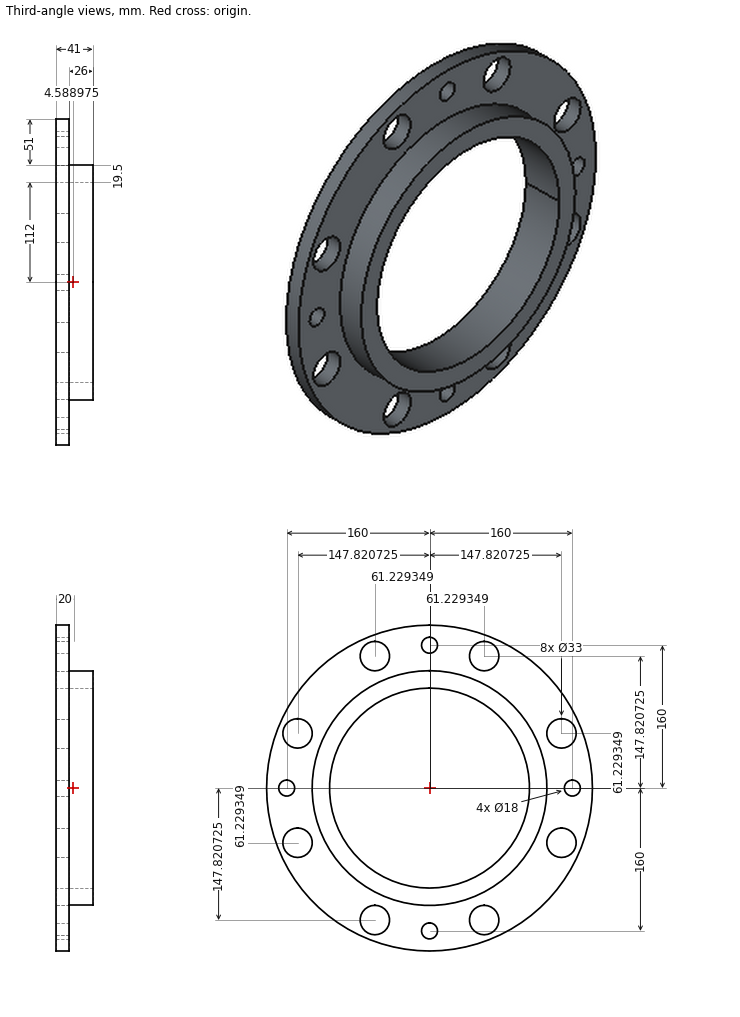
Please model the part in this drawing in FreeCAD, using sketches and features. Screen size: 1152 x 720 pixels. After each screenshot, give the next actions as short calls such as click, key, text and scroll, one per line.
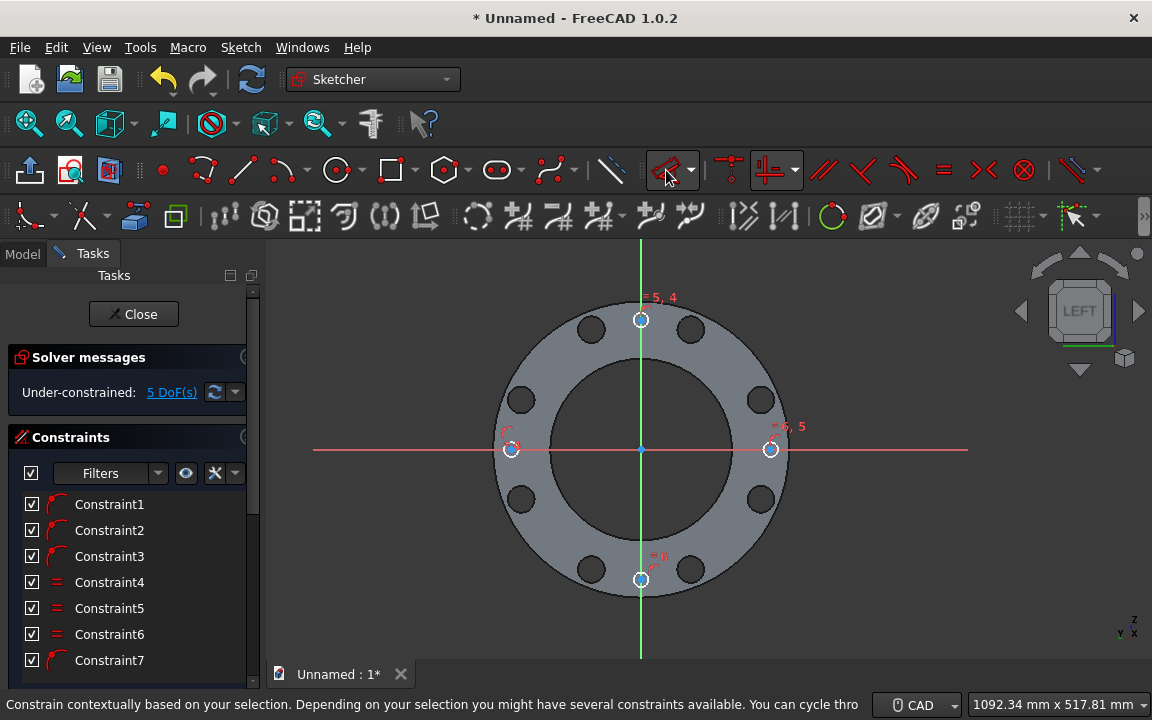
scroll(519, 450, up, 6)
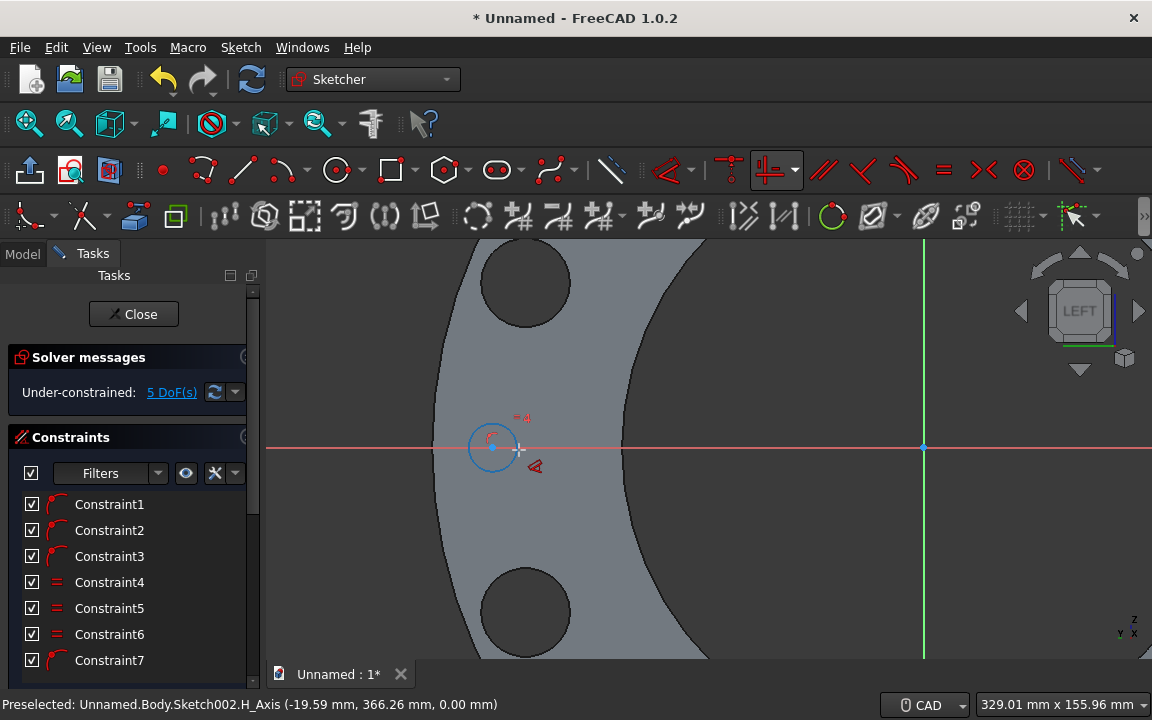
click(517, 448)
click(542, 475)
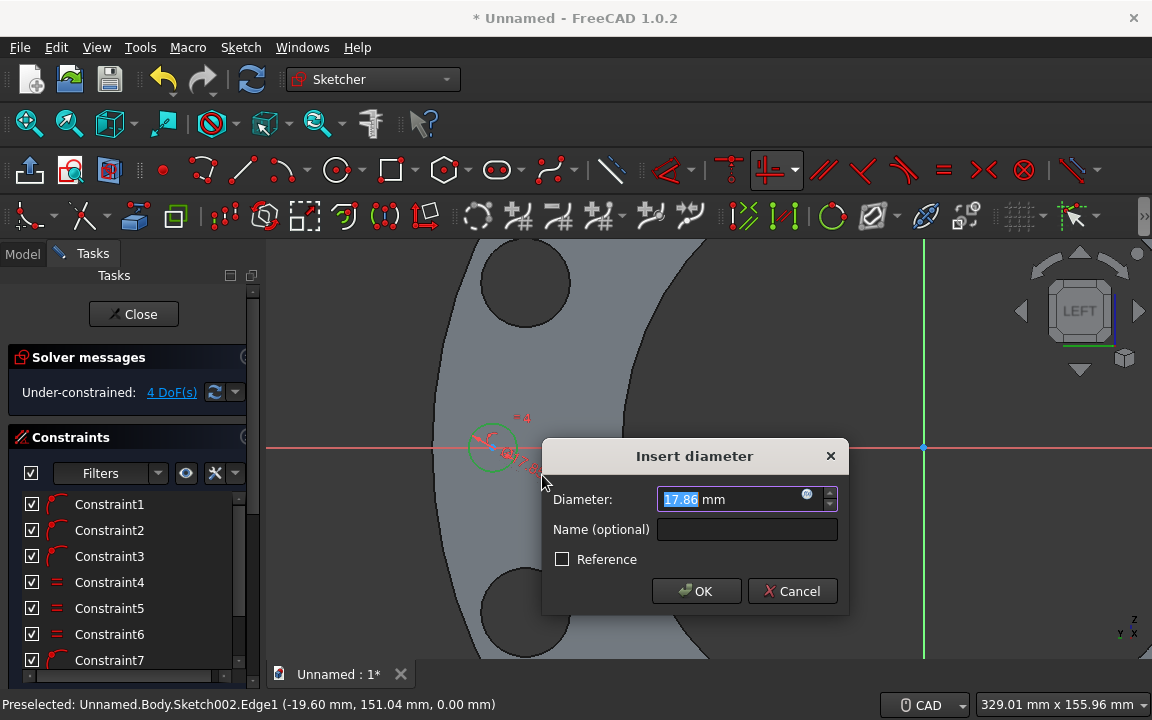
text(18)
key(Return)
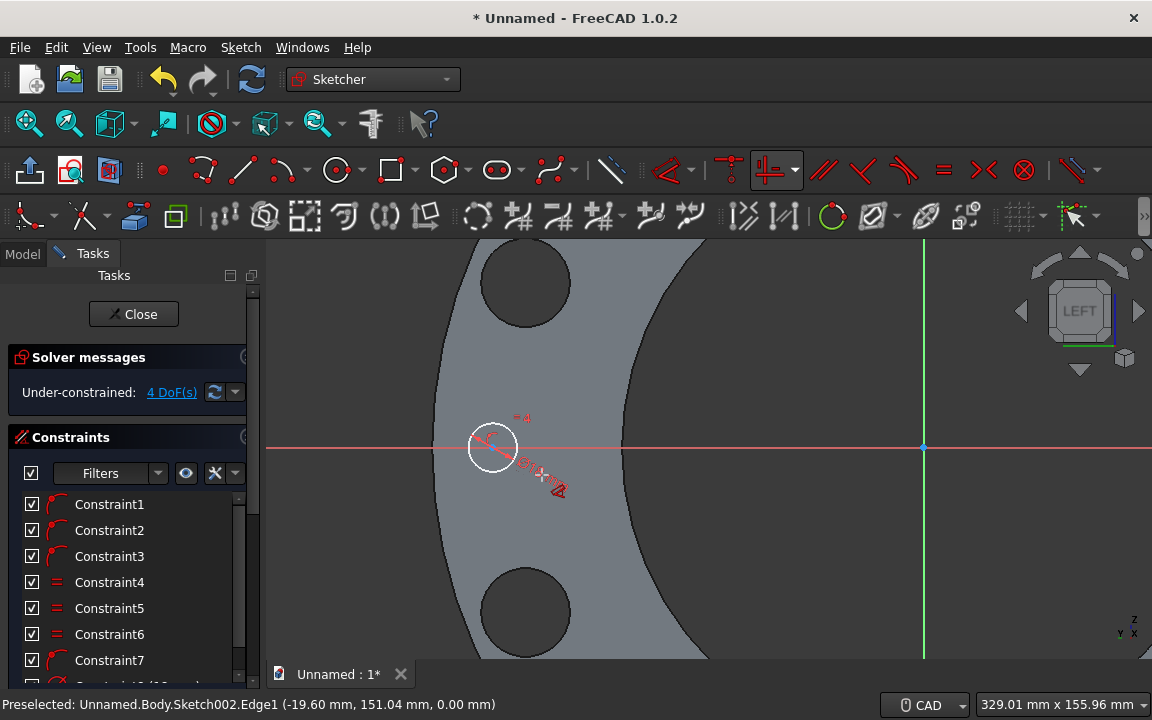
click(493, 448)
click(708, 482)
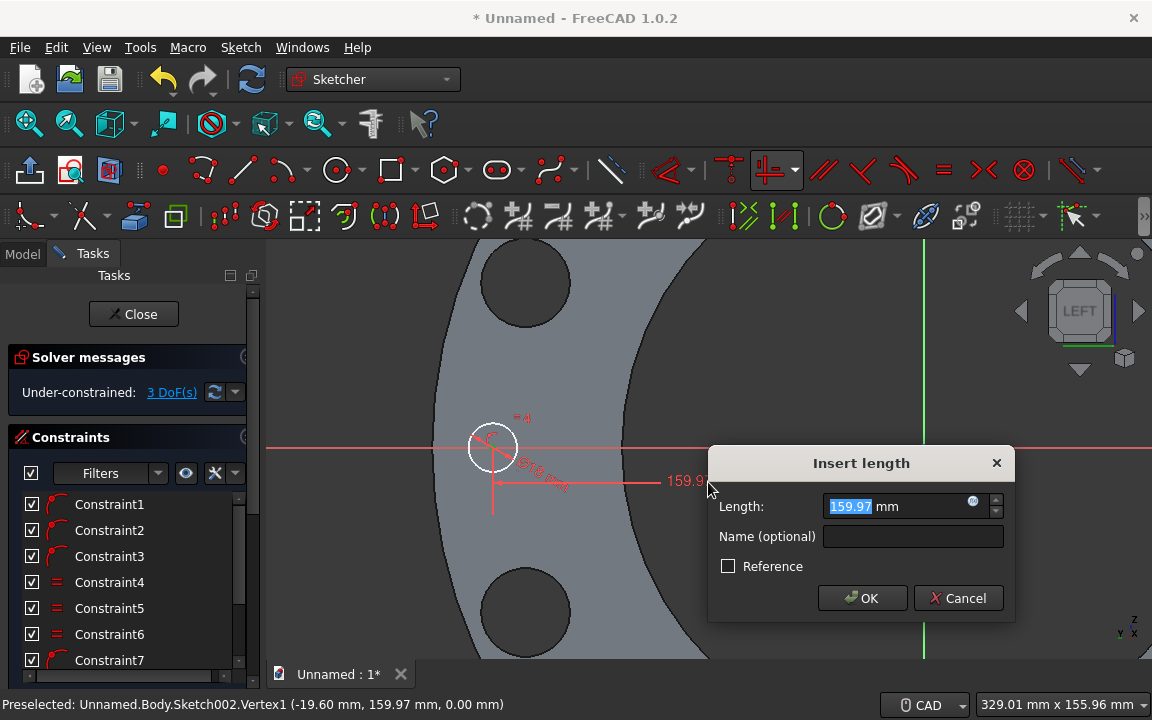
text(160)
key(Return)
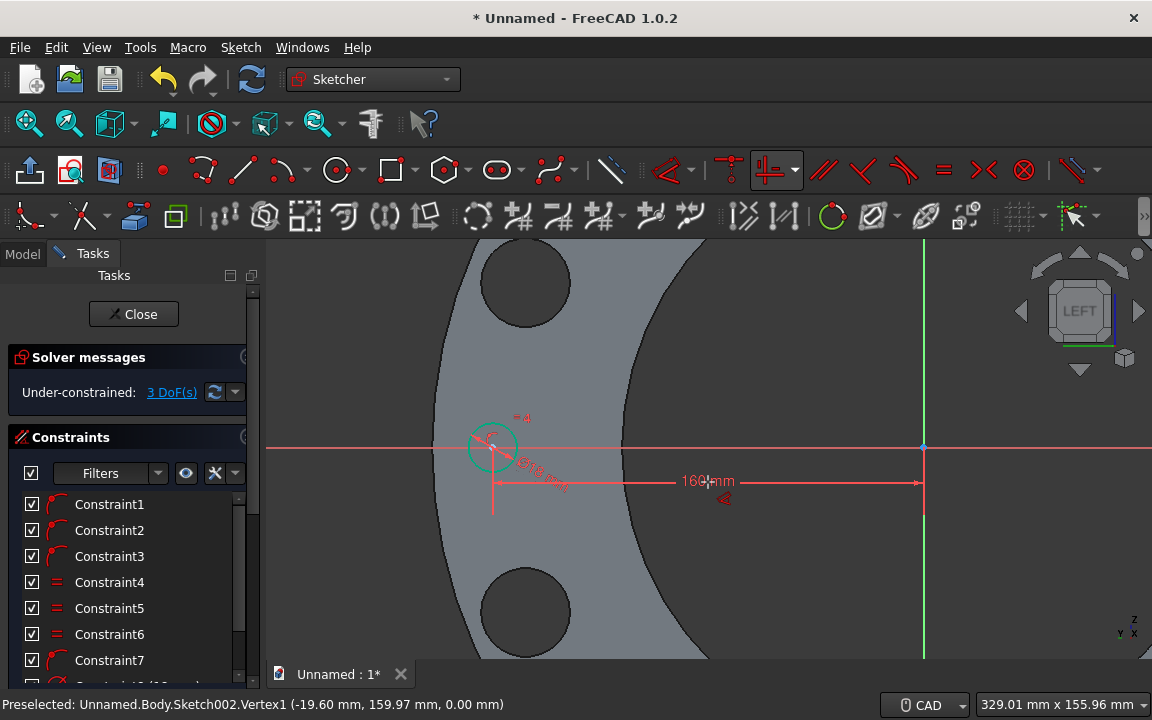
scroll(518, 450, down, 6)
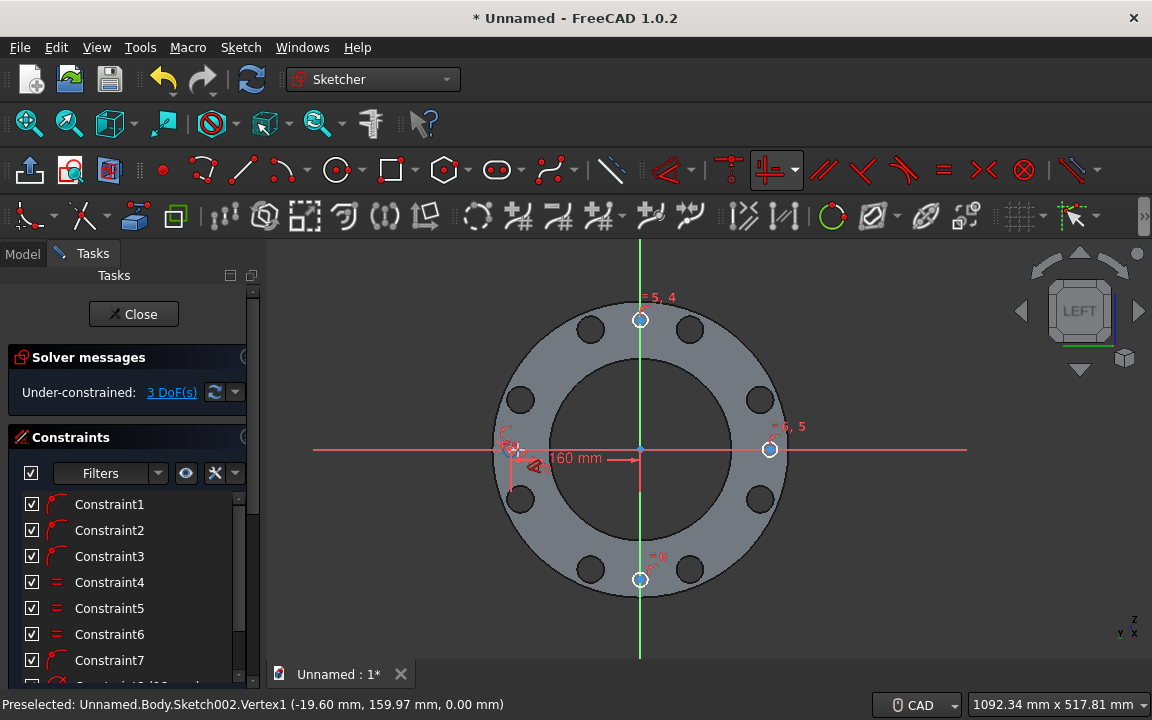
click(640, 320)
click(674, 385)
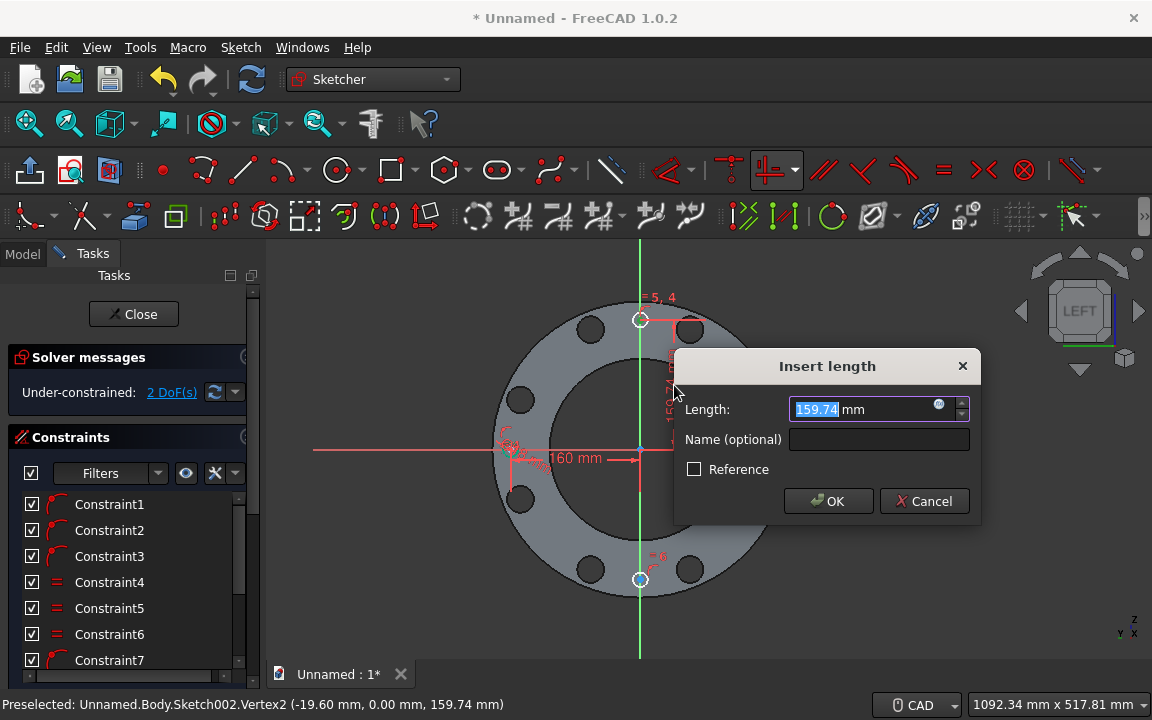
text(160)
key(Return)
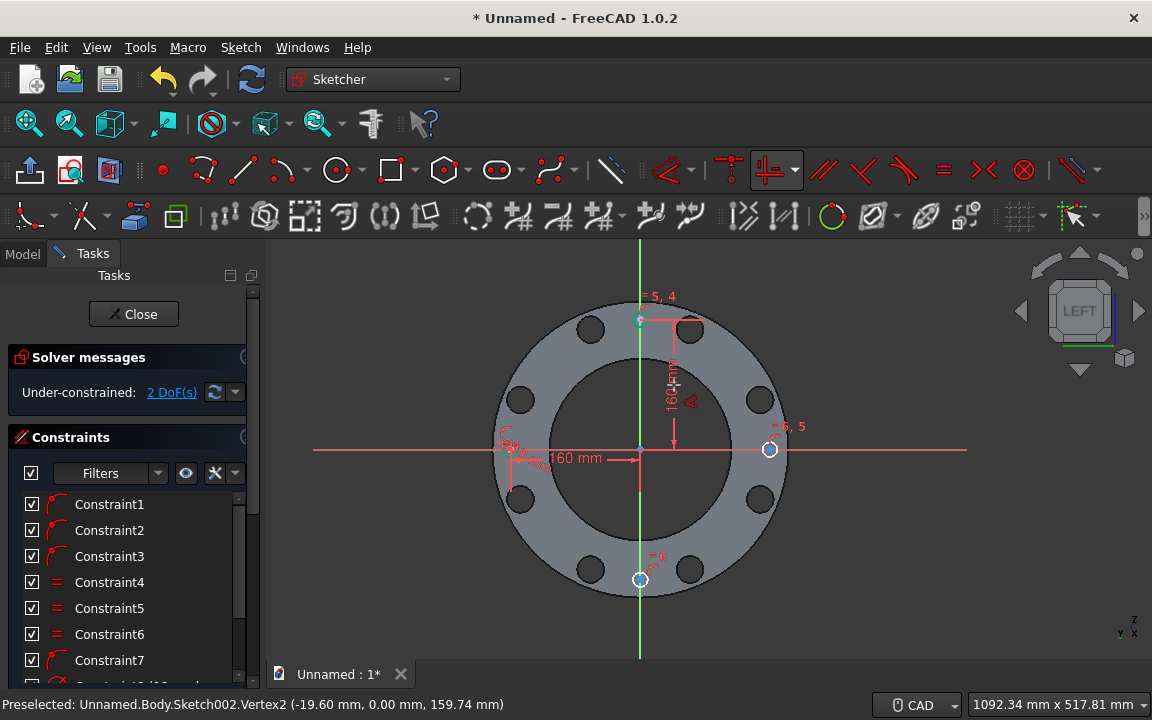
click(770, 450)
click(705, 484)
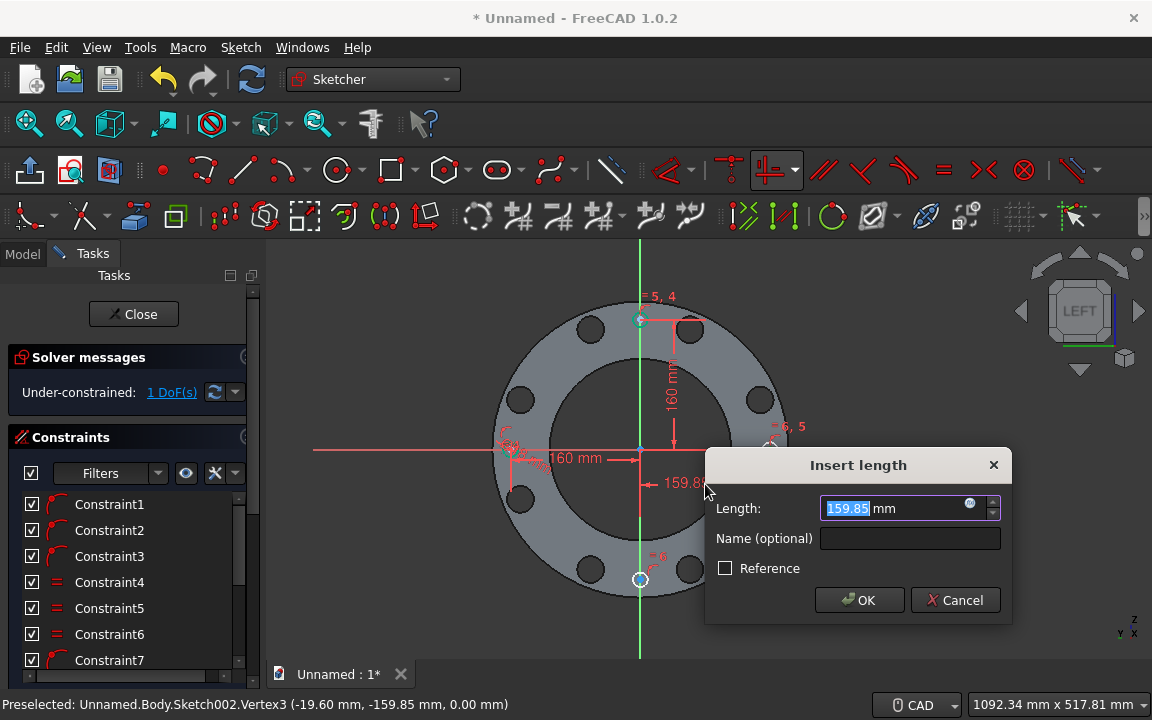
text(160)
key(Return)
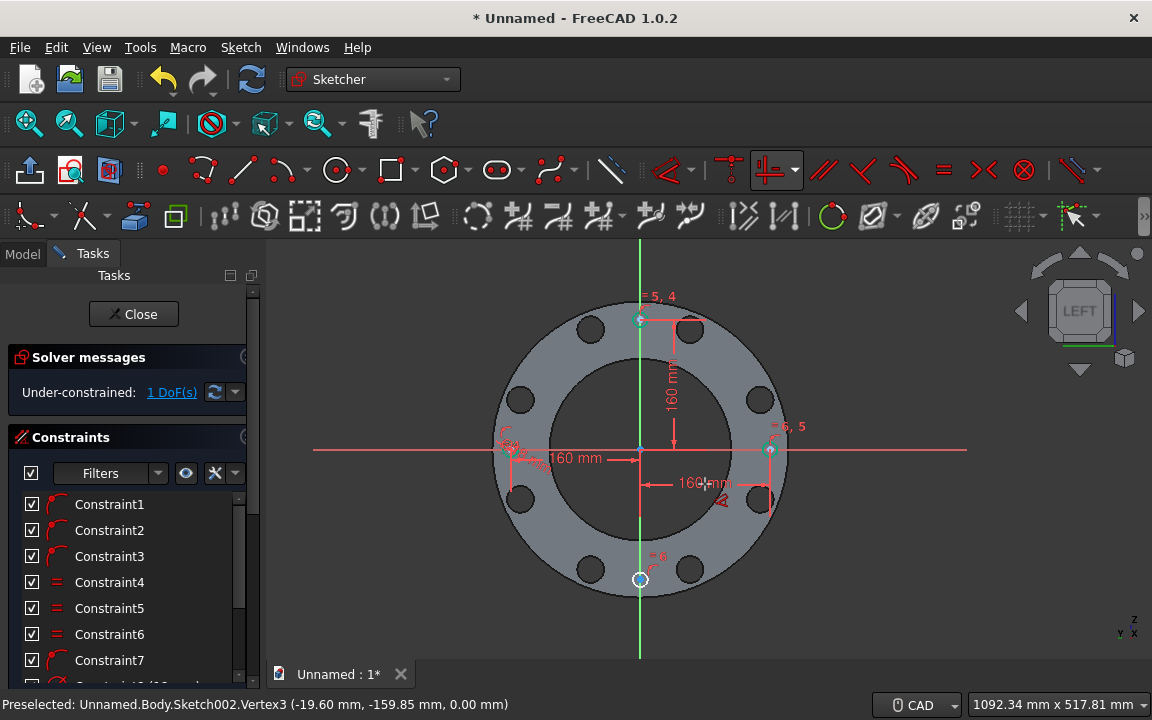
click(640, 580)
click(674, 515)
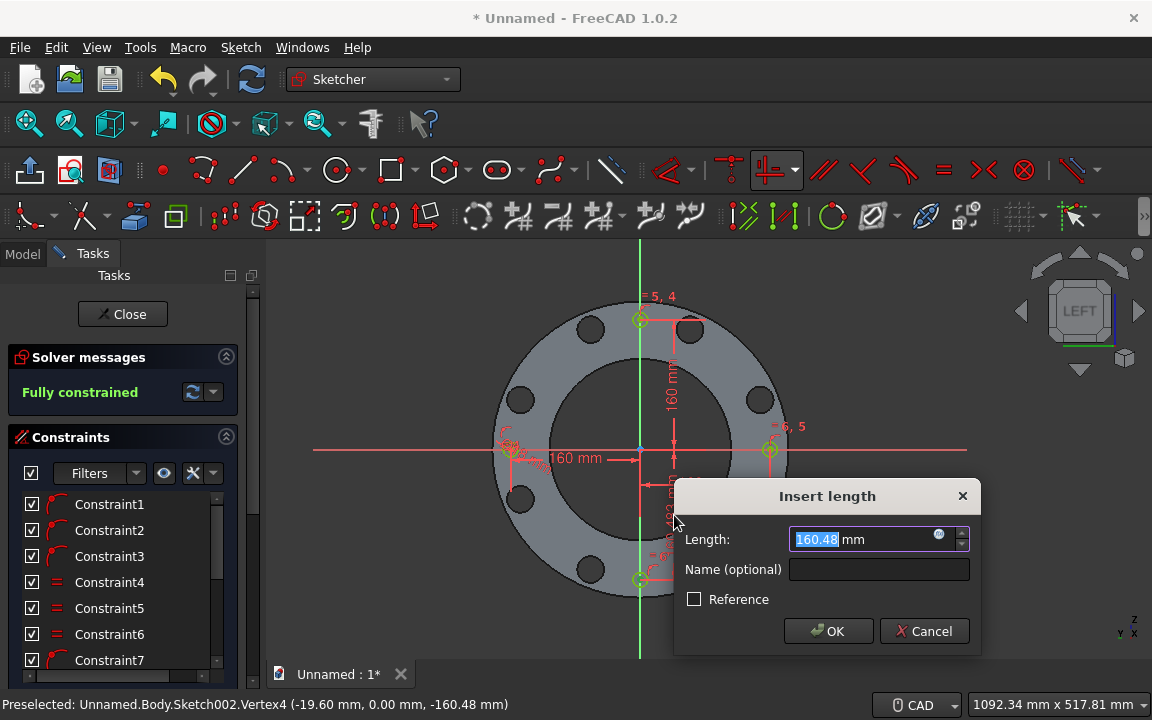
text(160)
key(Return)
key(Escape)